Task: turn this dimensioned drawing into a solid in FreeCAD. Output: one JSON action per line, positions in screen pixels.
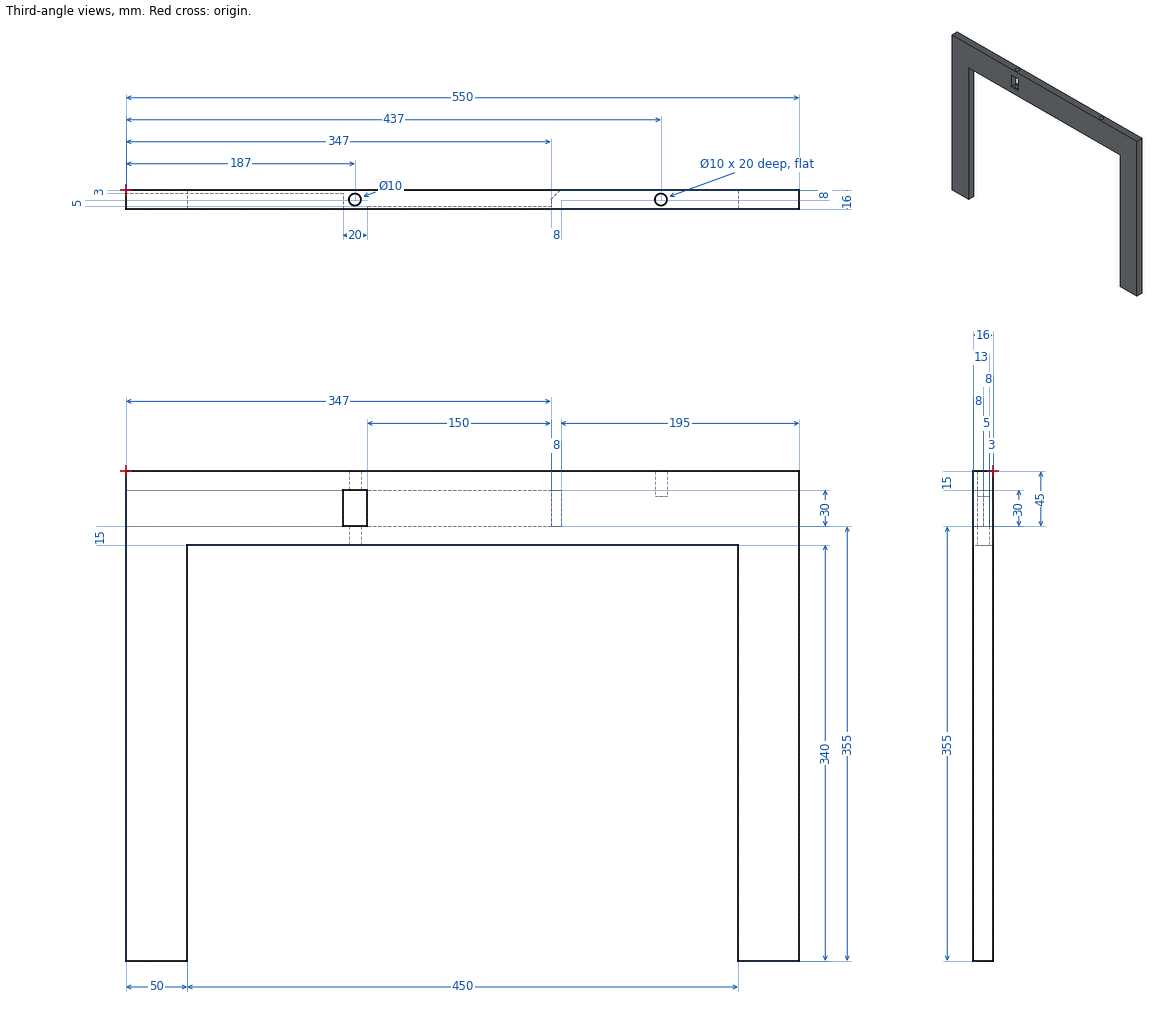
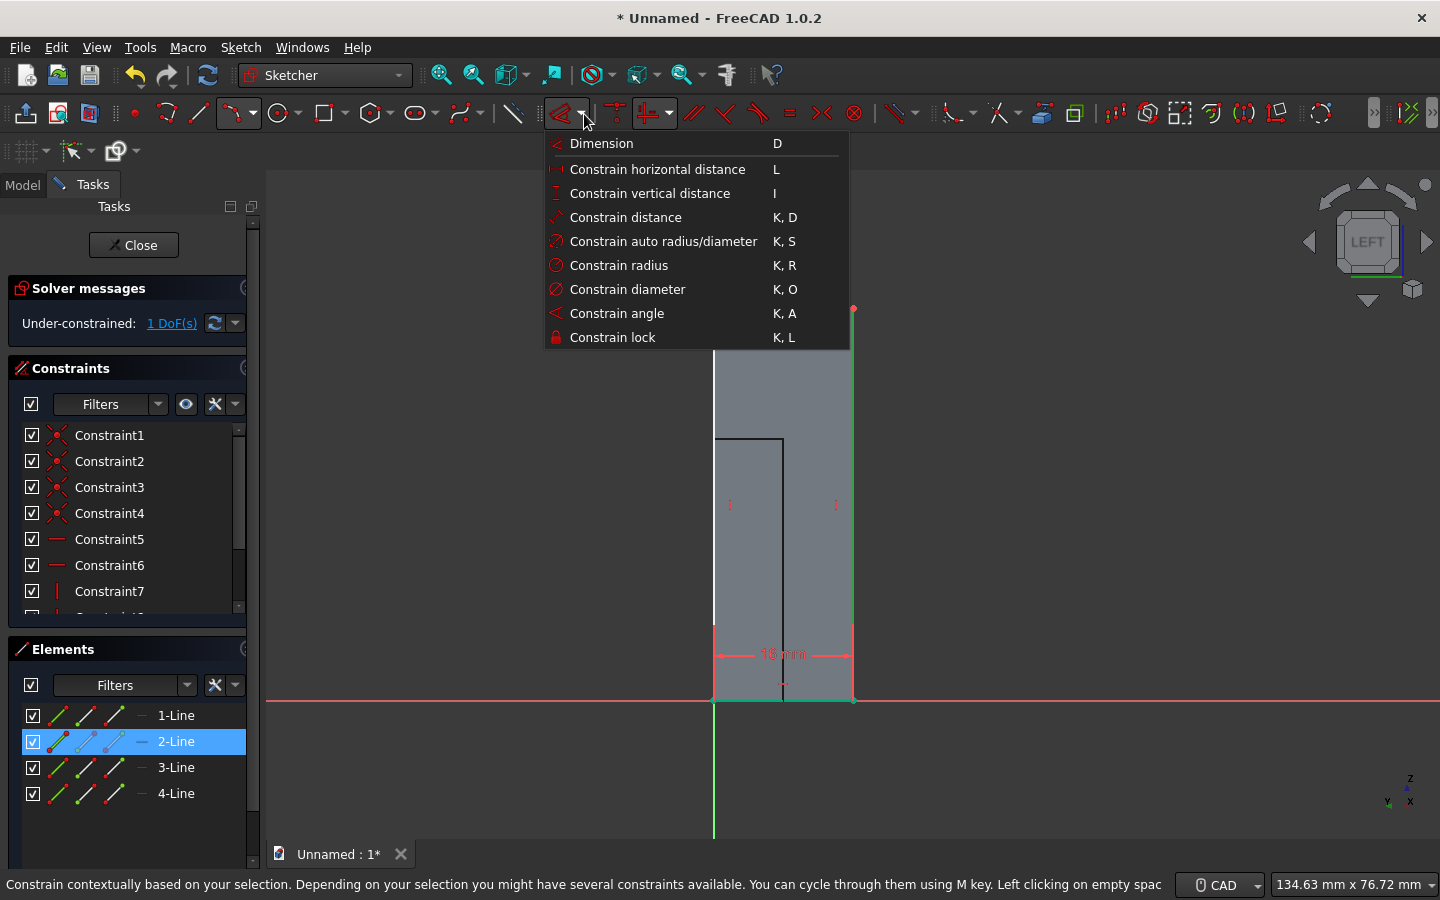
{"action": "left_click", "coordinate": [697, 193]}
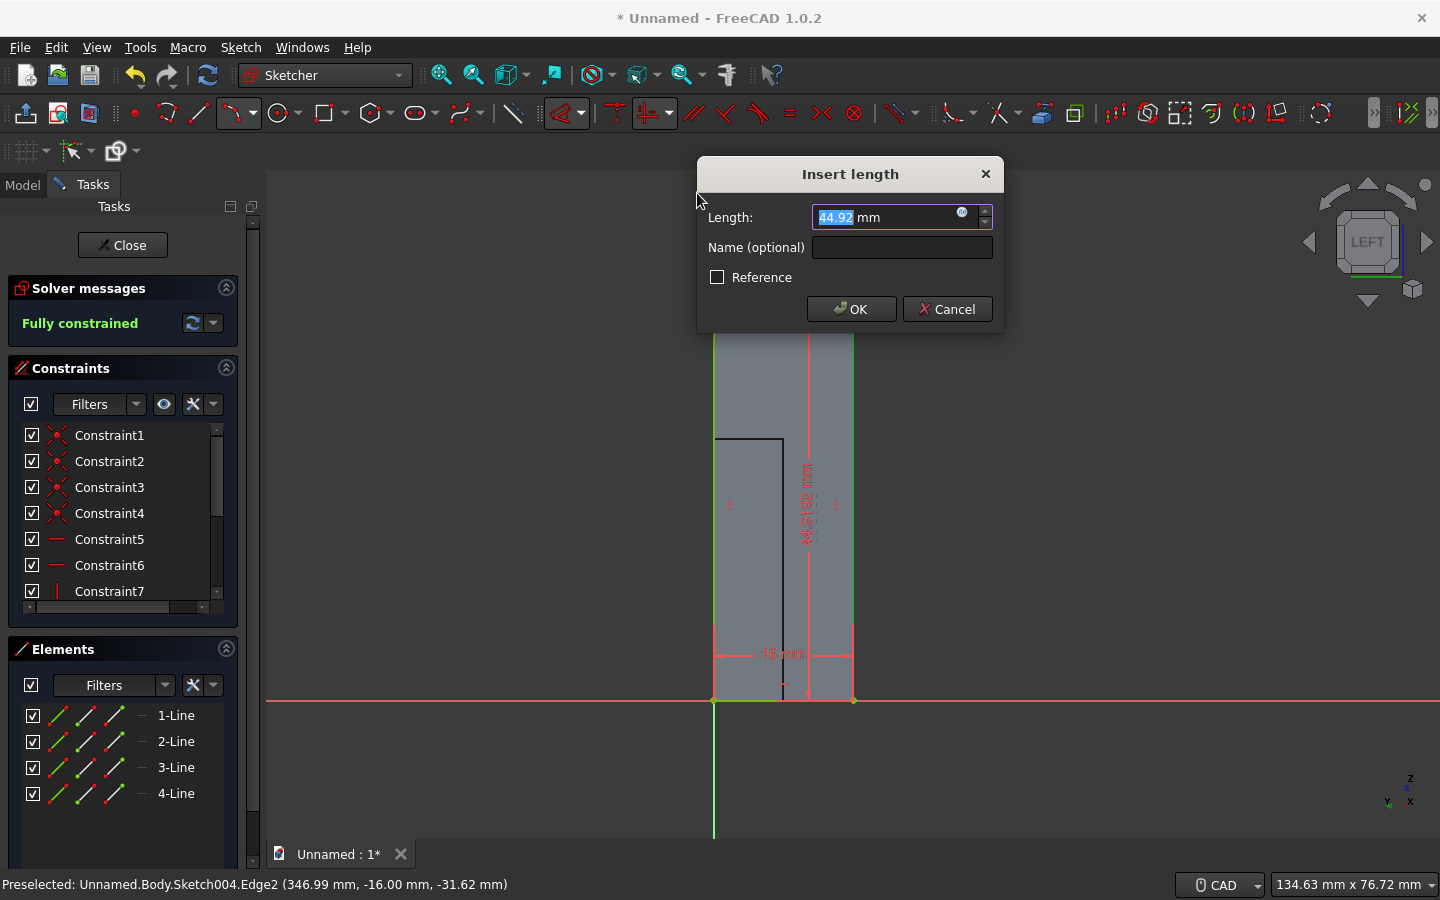
{"action": "type", "text": "45"}
{"action": "key", "text": "Return"}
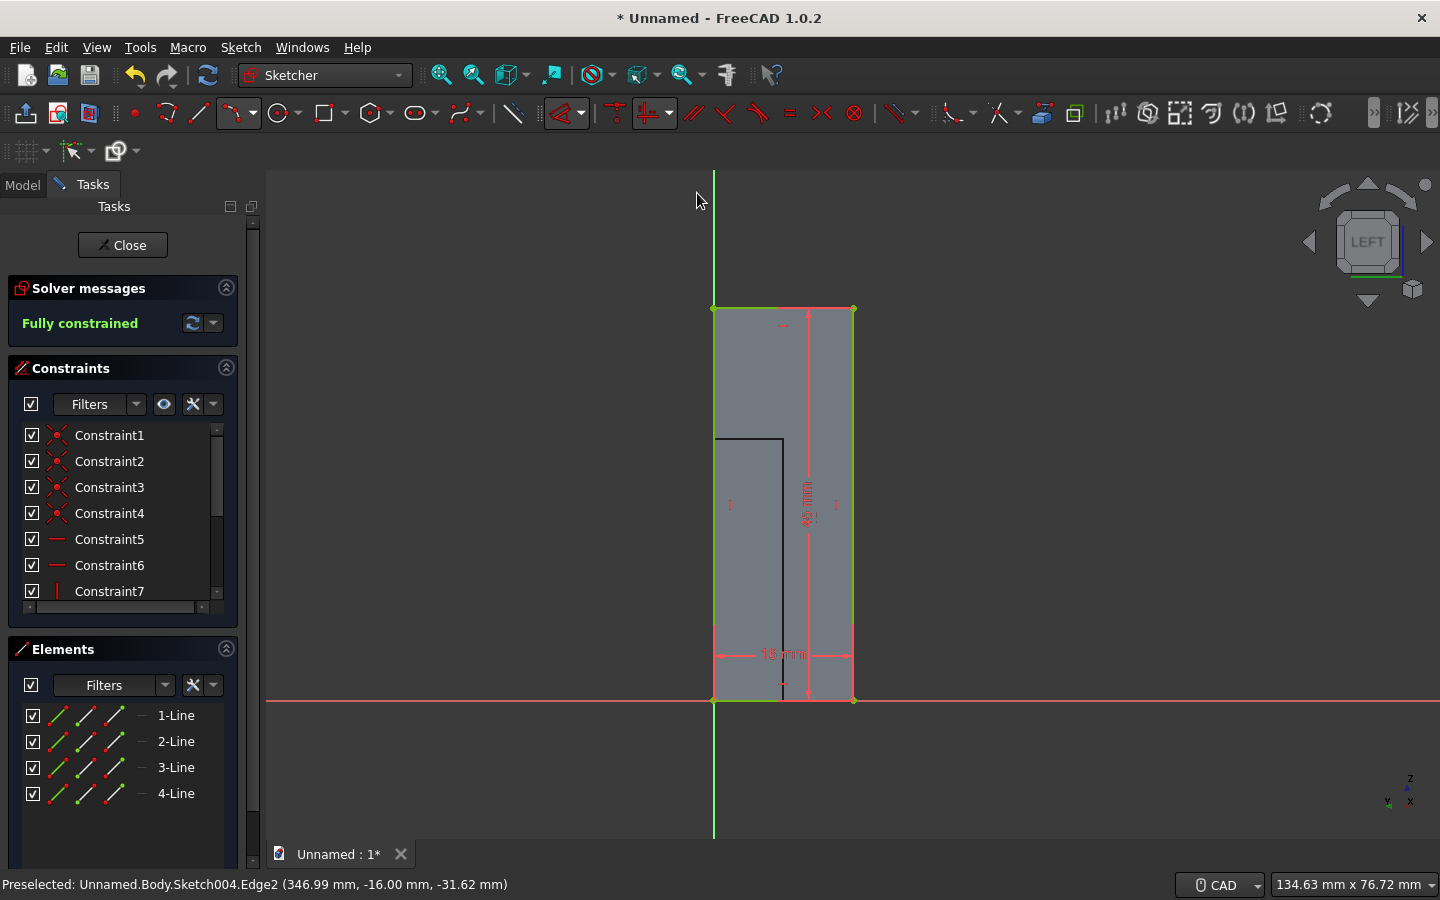
{"action": "left_click", "coordinate": [123, 245]}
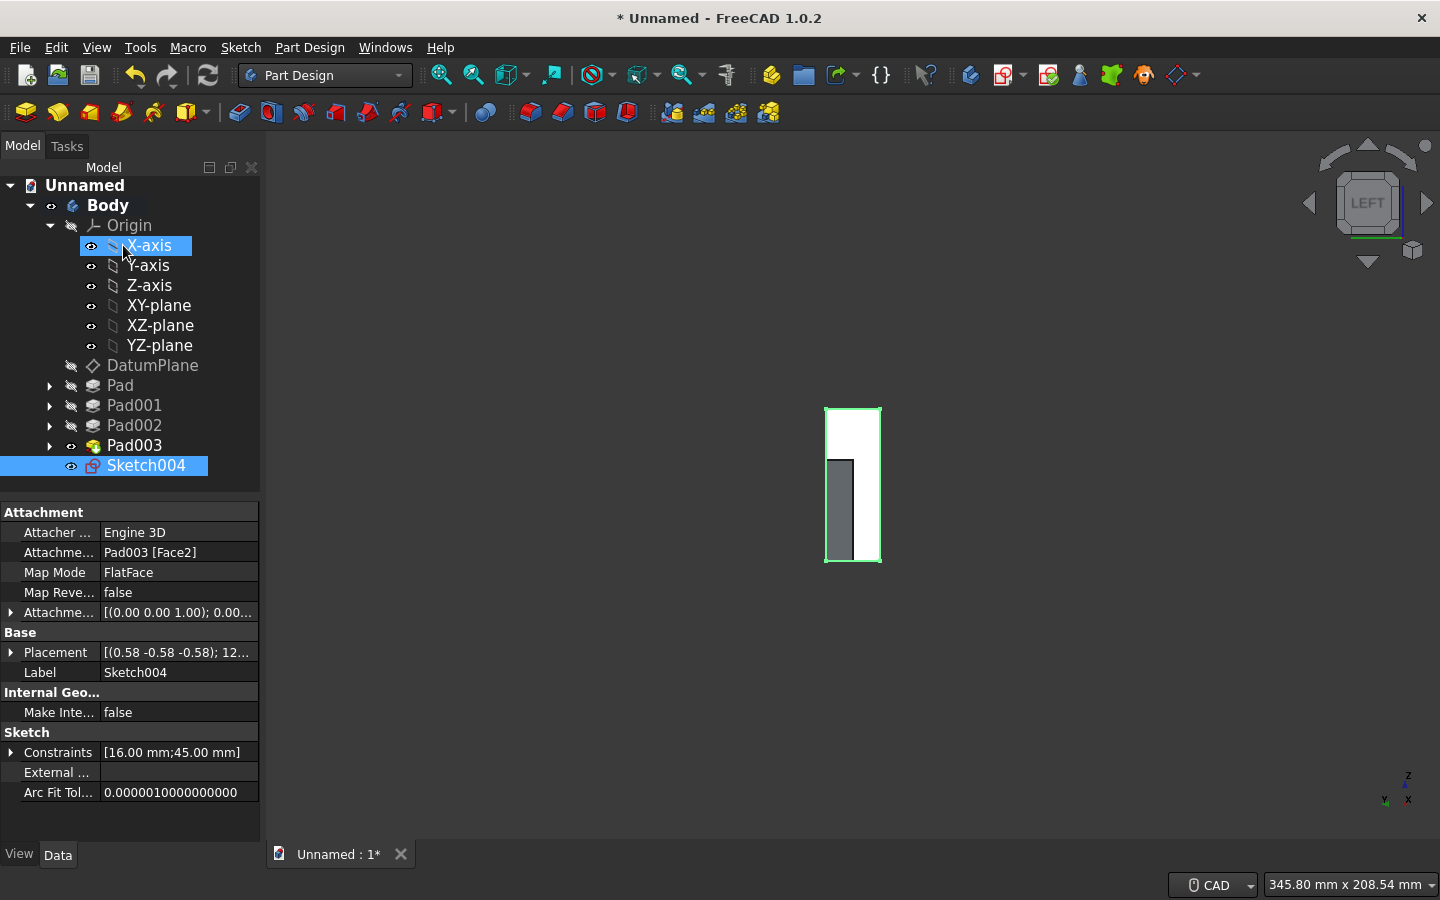
{"action": "left_click", "coordinate": [26, 112]}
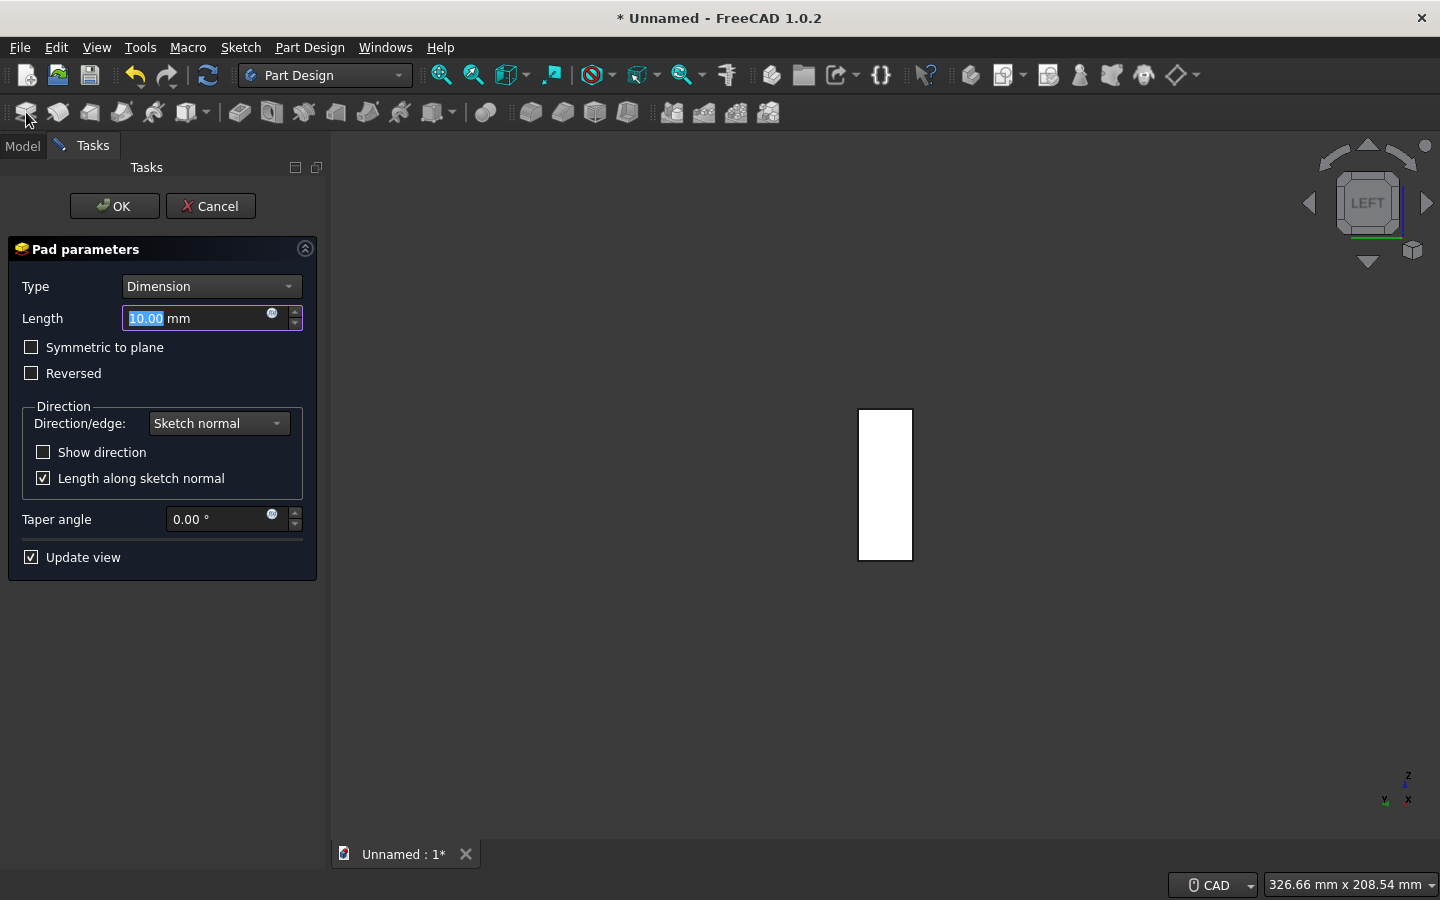
{"action": "type", "text": "347"}
{"action": "key", "text": "Tab"}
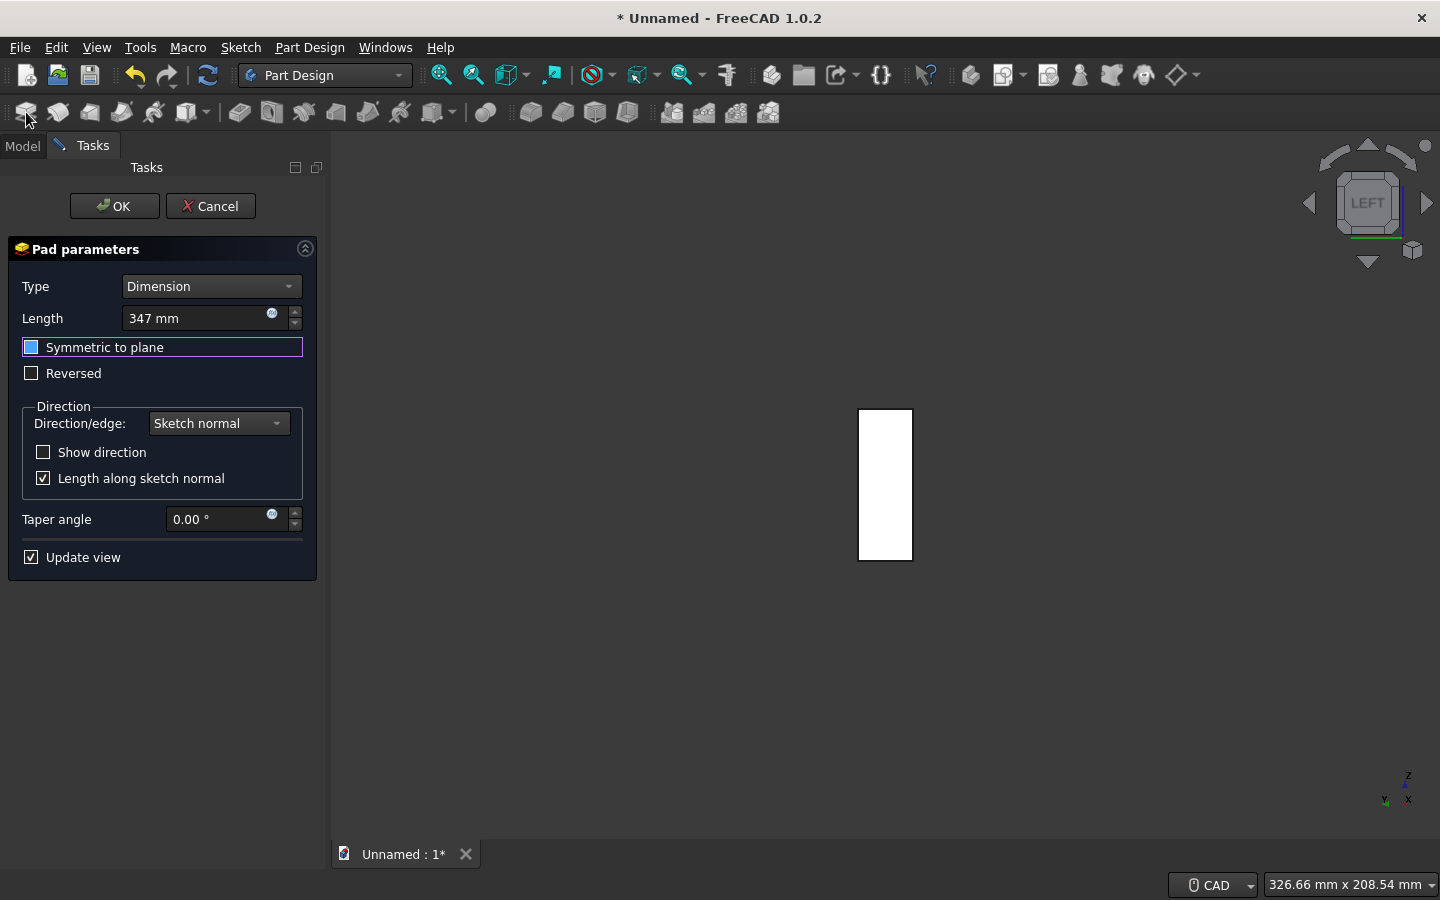
{"action": "left_click", "coordinate": [115, 206]}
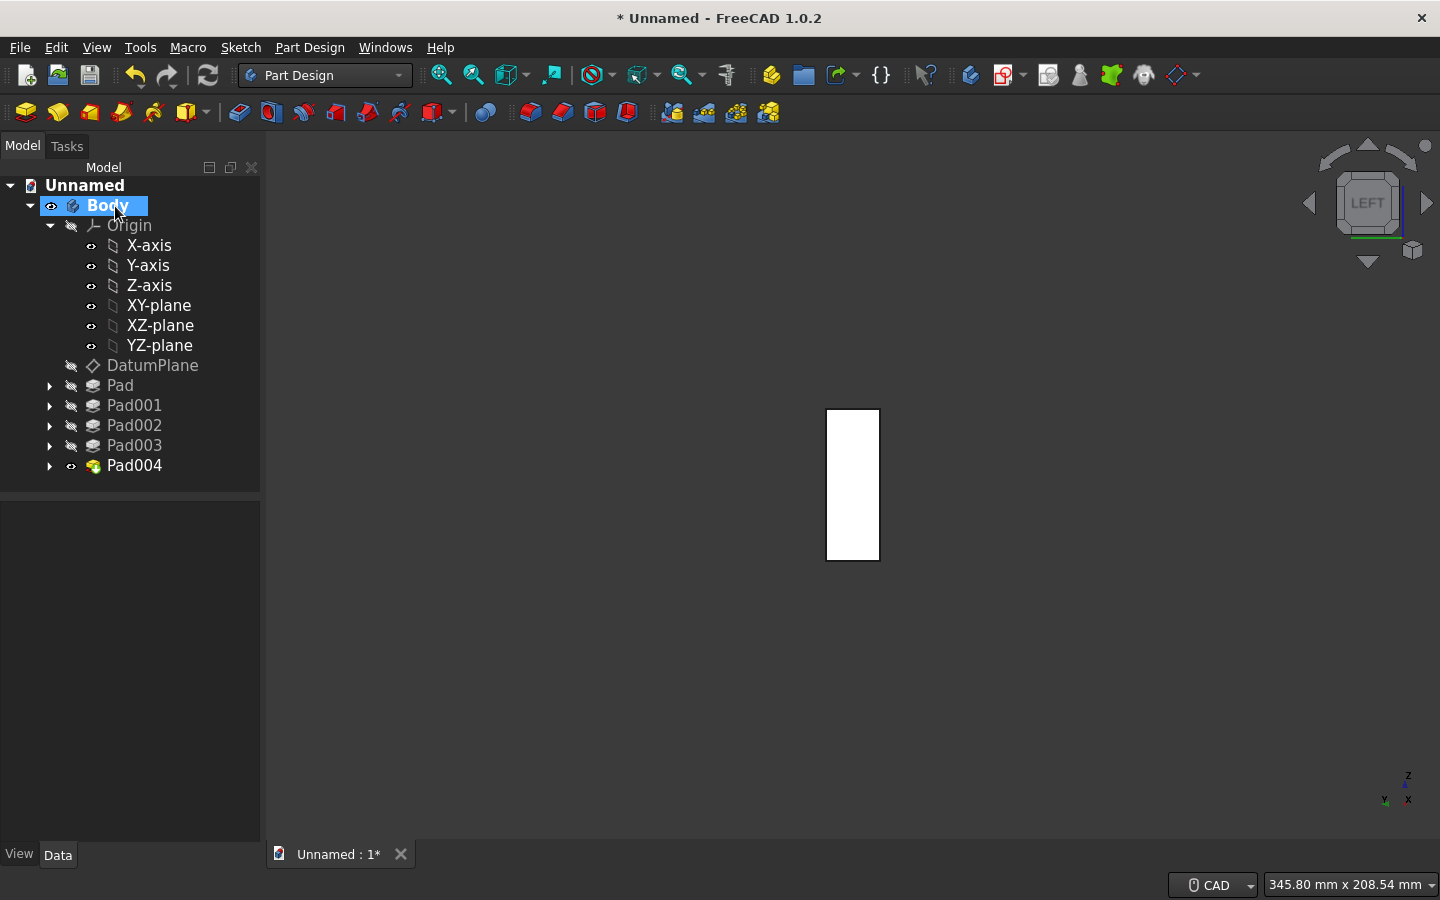
{"action": "left_click", "coordinate": [442, 76]}